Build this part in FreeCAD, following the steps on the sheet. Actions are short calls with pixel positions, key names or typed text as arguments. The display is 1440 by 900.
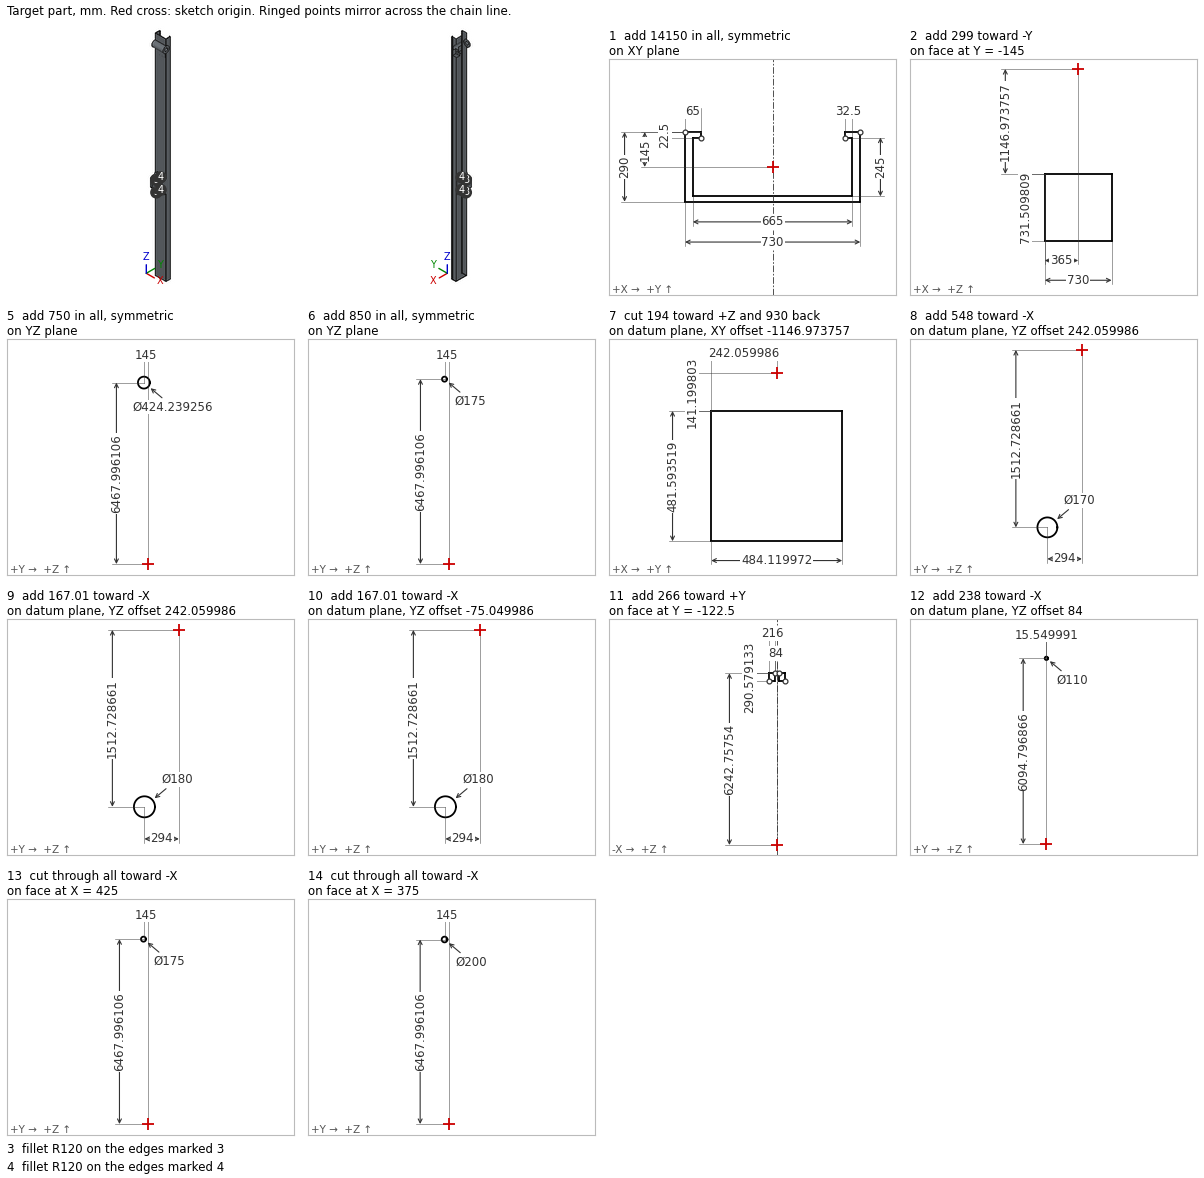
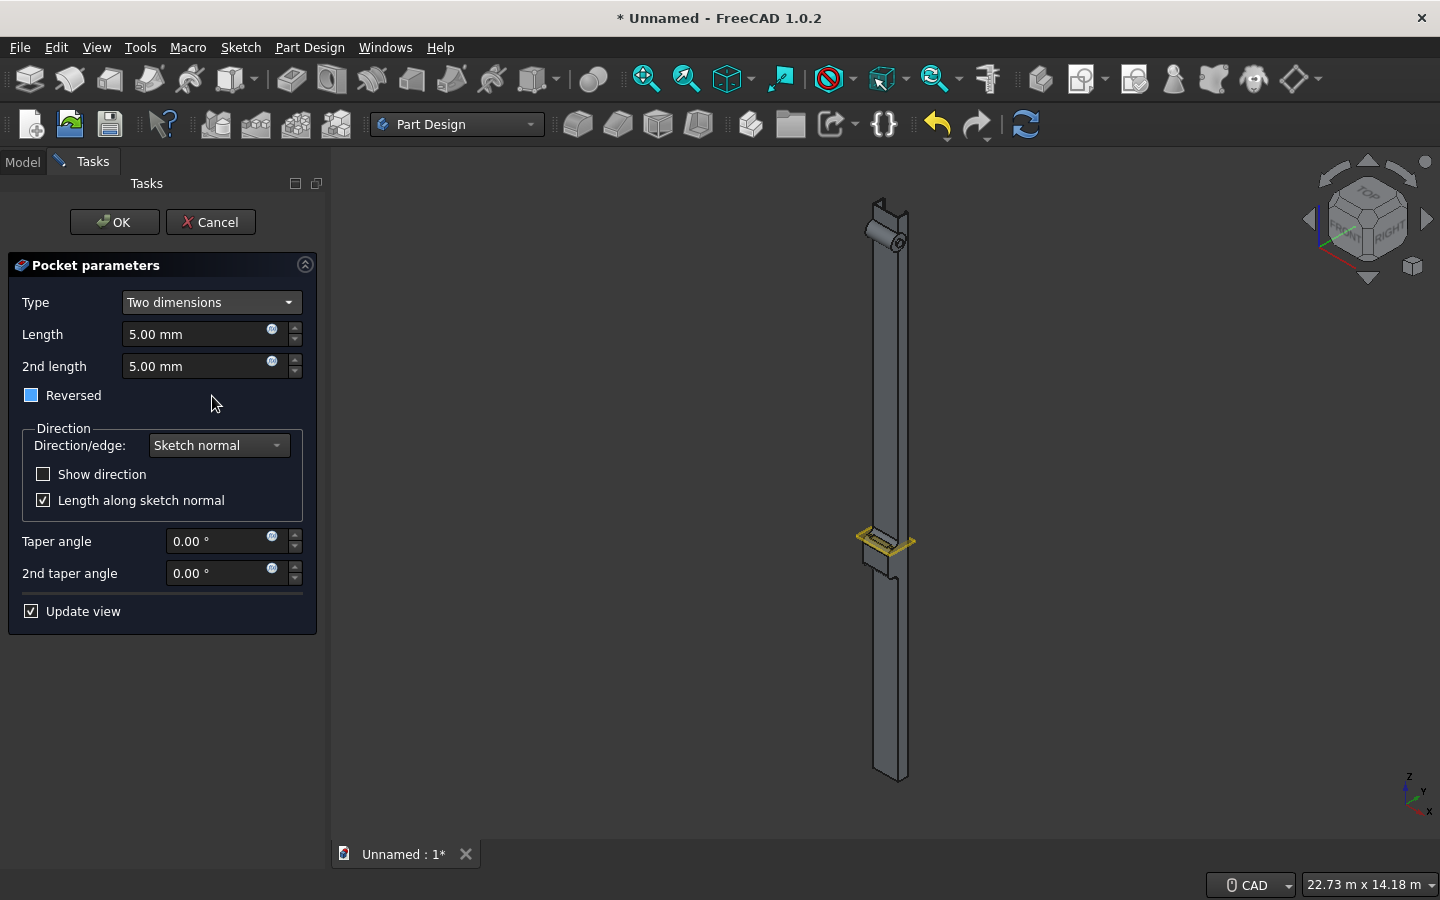
triple_click(204, 334)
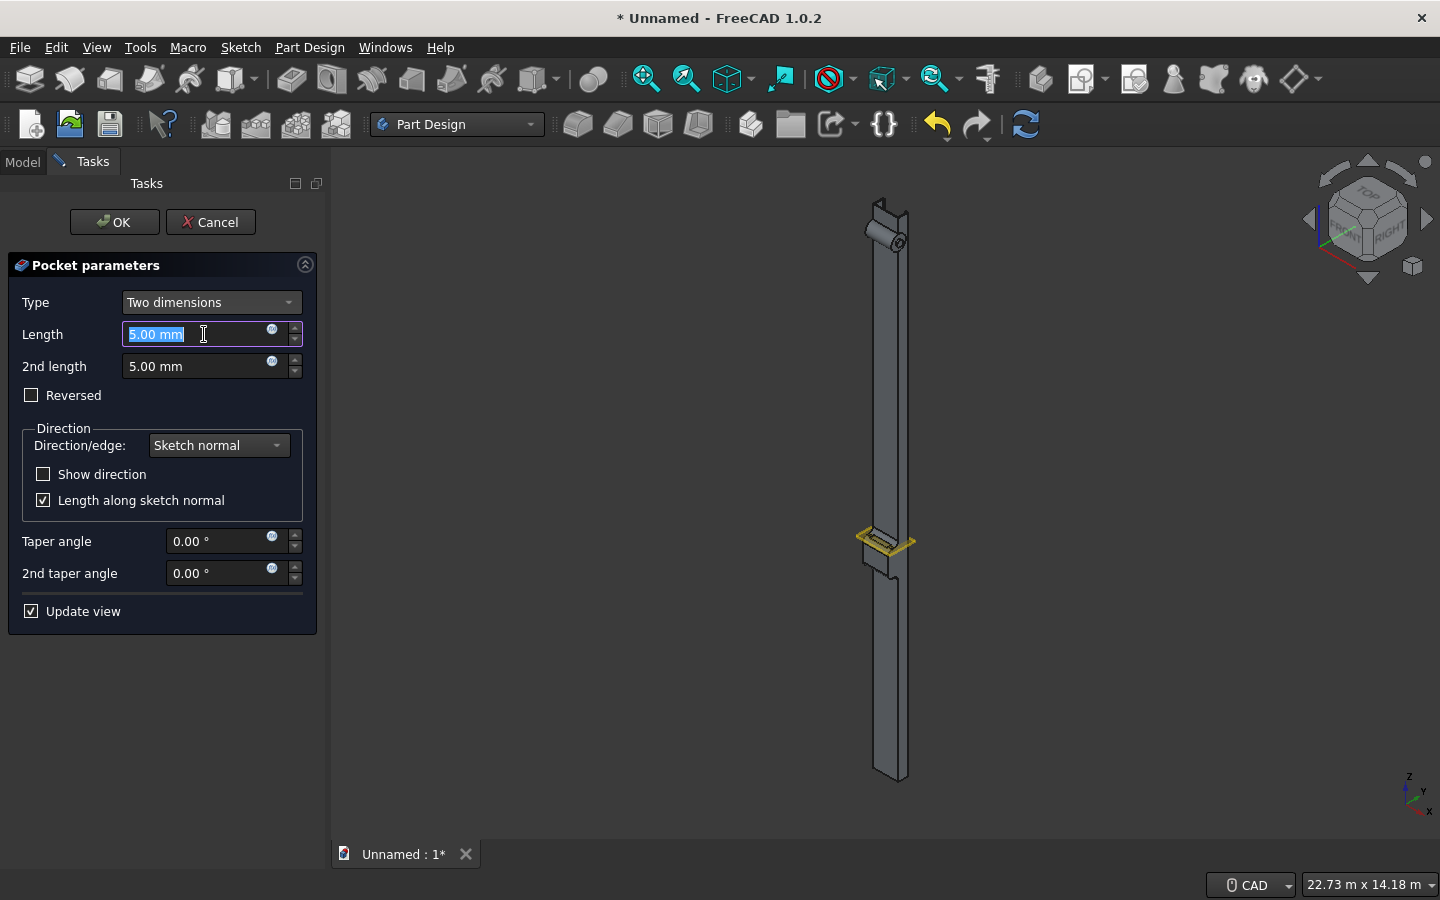
text(194)
key(Tab)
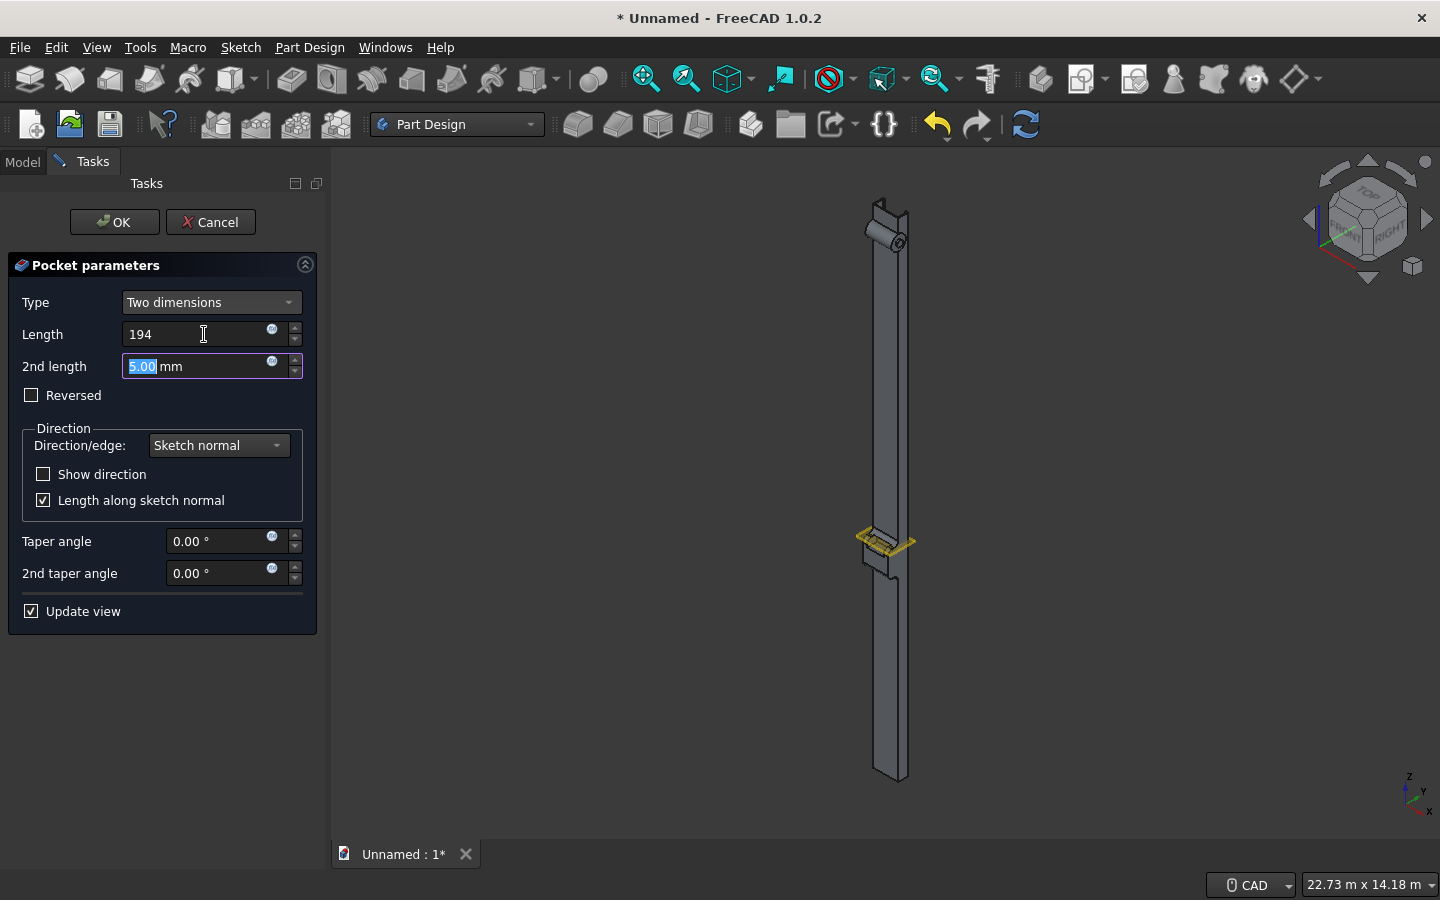
text(930)
key(Tab)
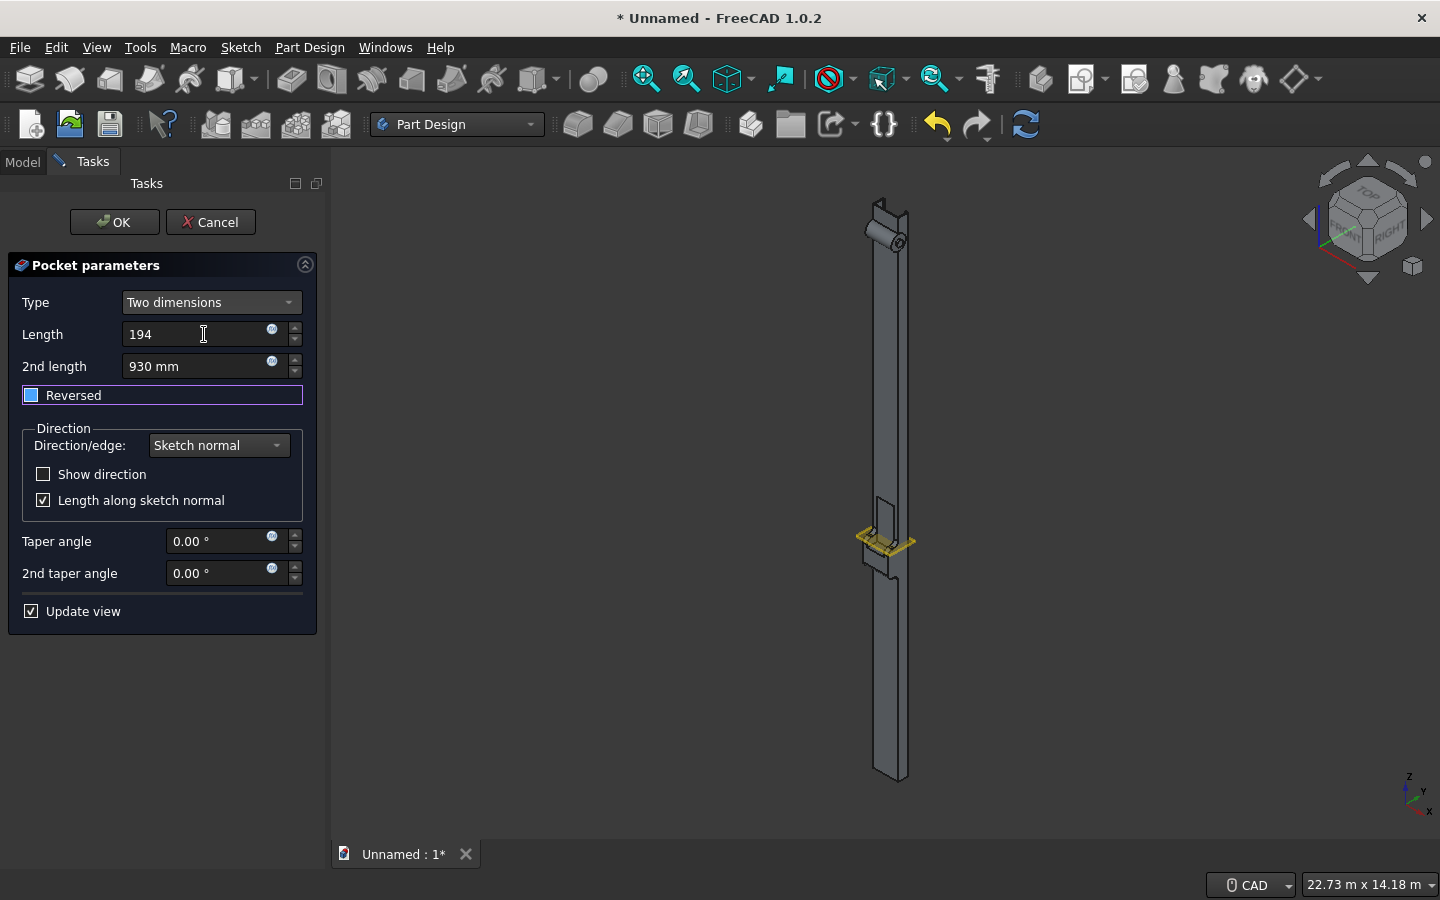
click(30, 395)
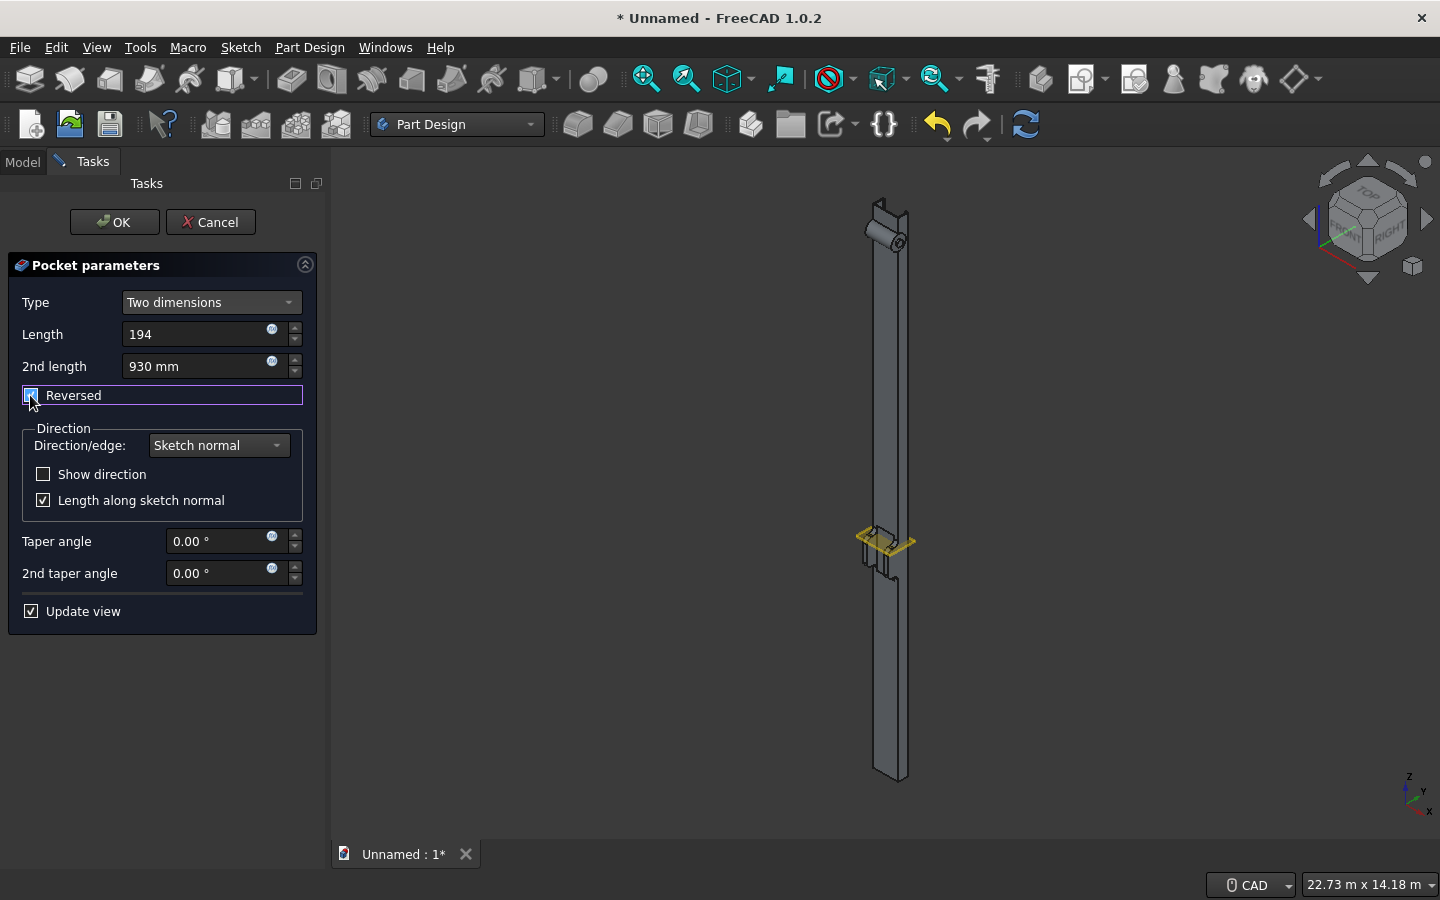
click(115, 222)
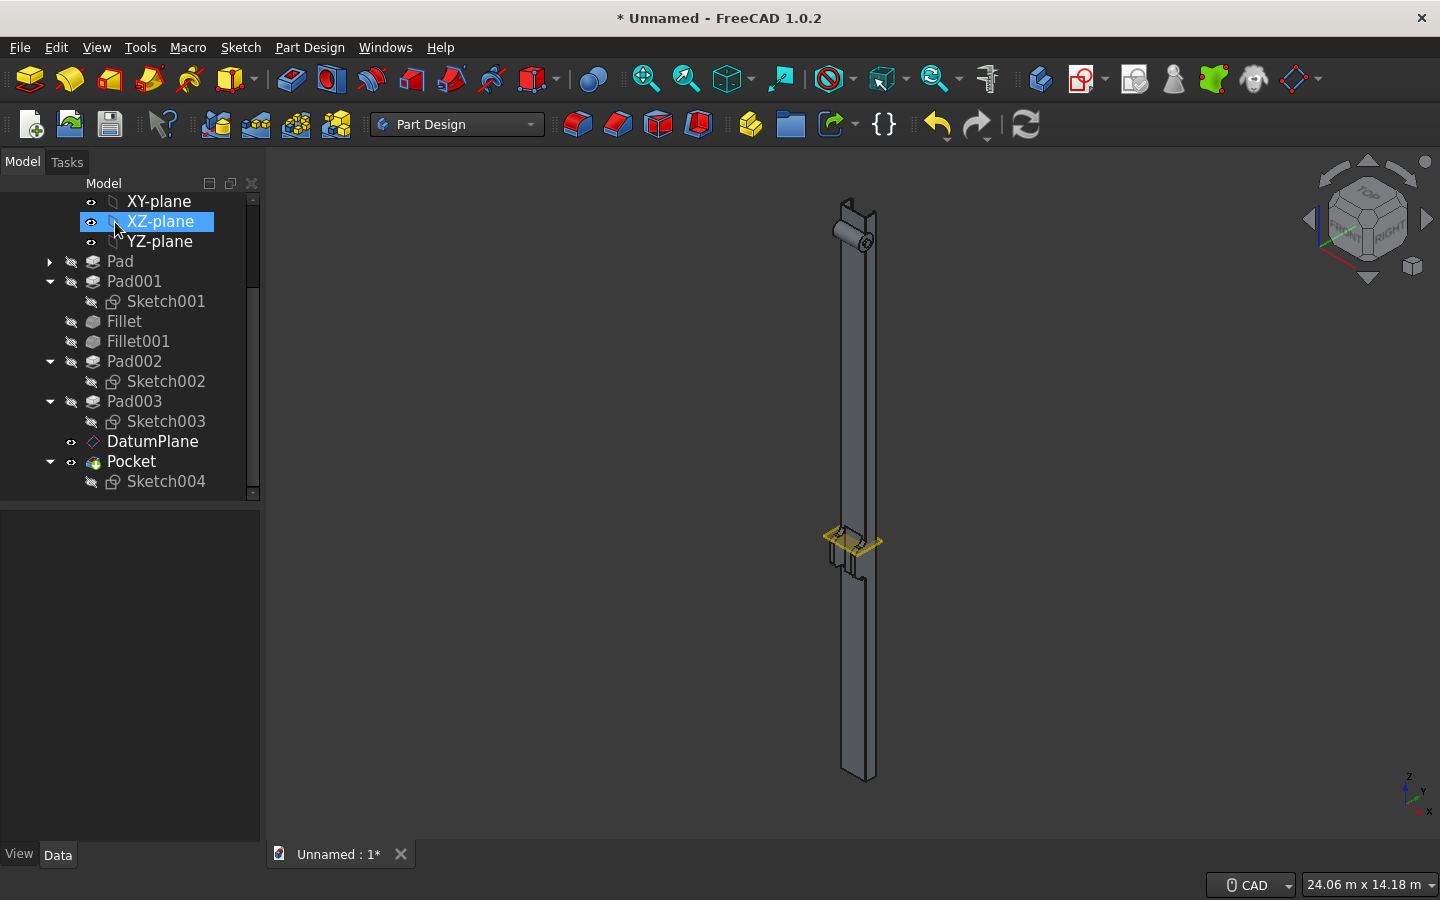
click(116, 442)
key(space)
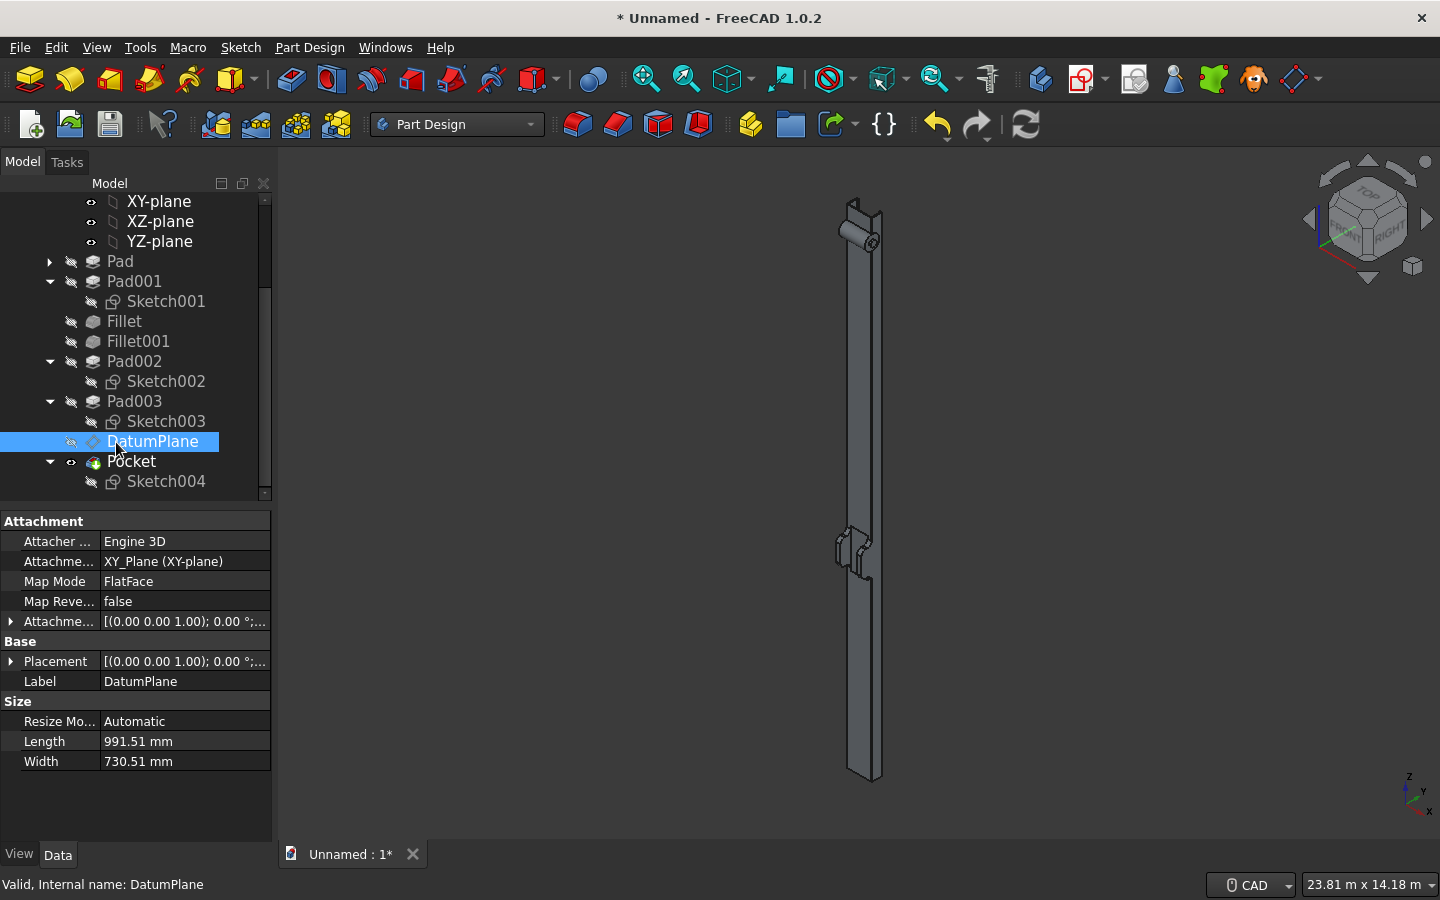
scroll(160, 337, down, 3)